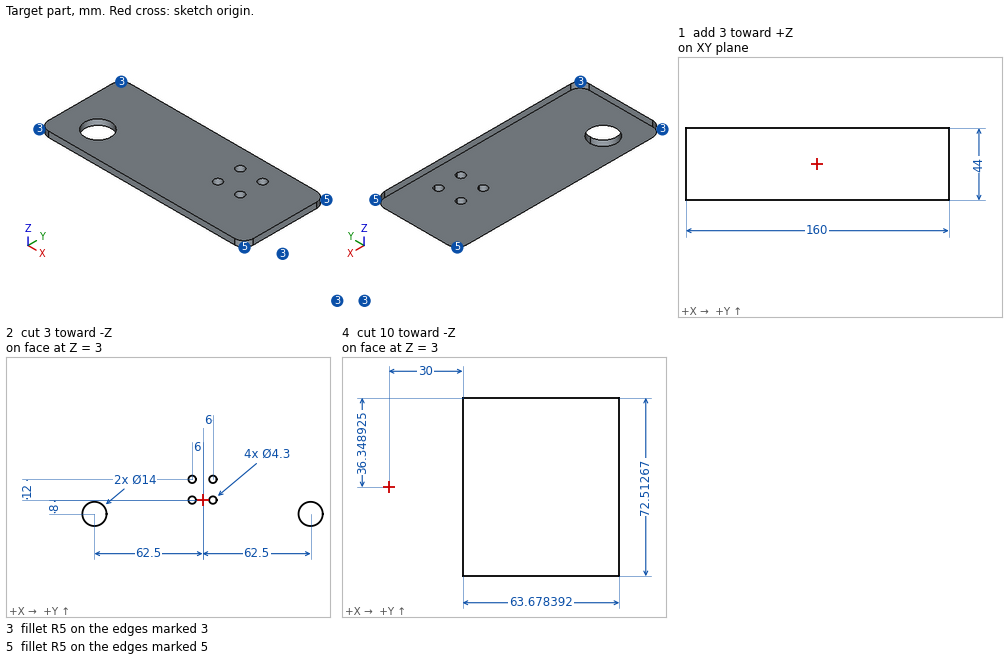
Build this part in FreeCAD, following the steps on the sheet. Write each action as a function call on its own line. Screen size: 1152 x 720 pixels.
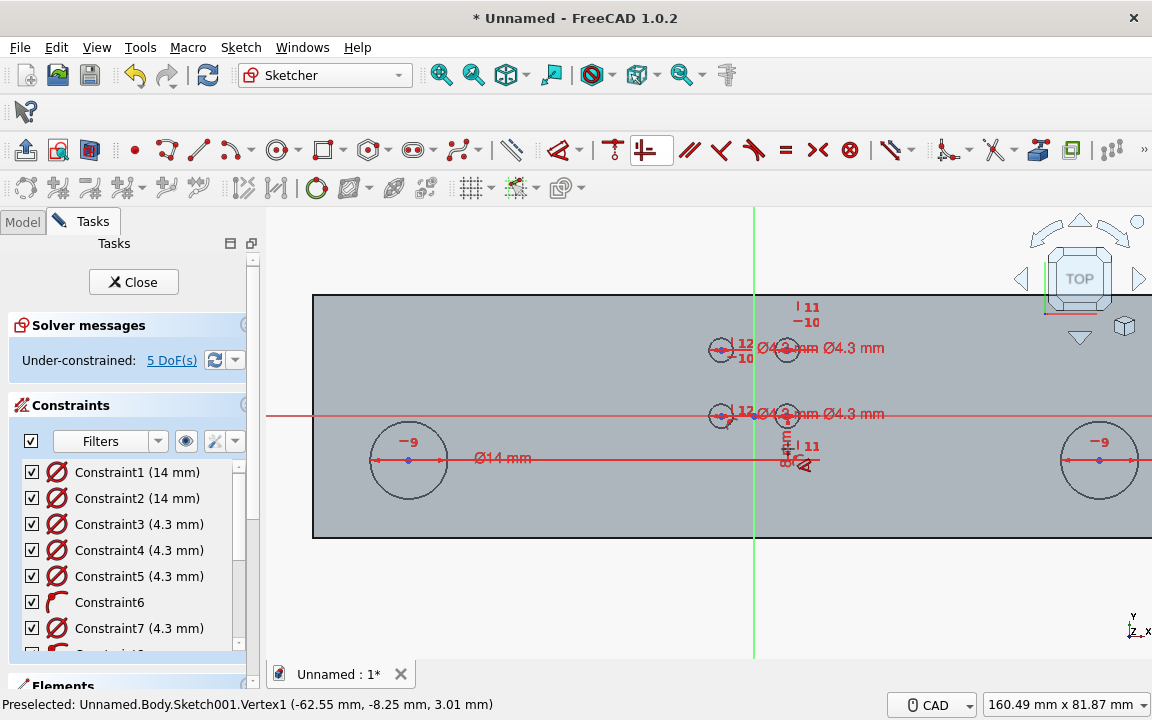
click(721, 350)
click(738, 316)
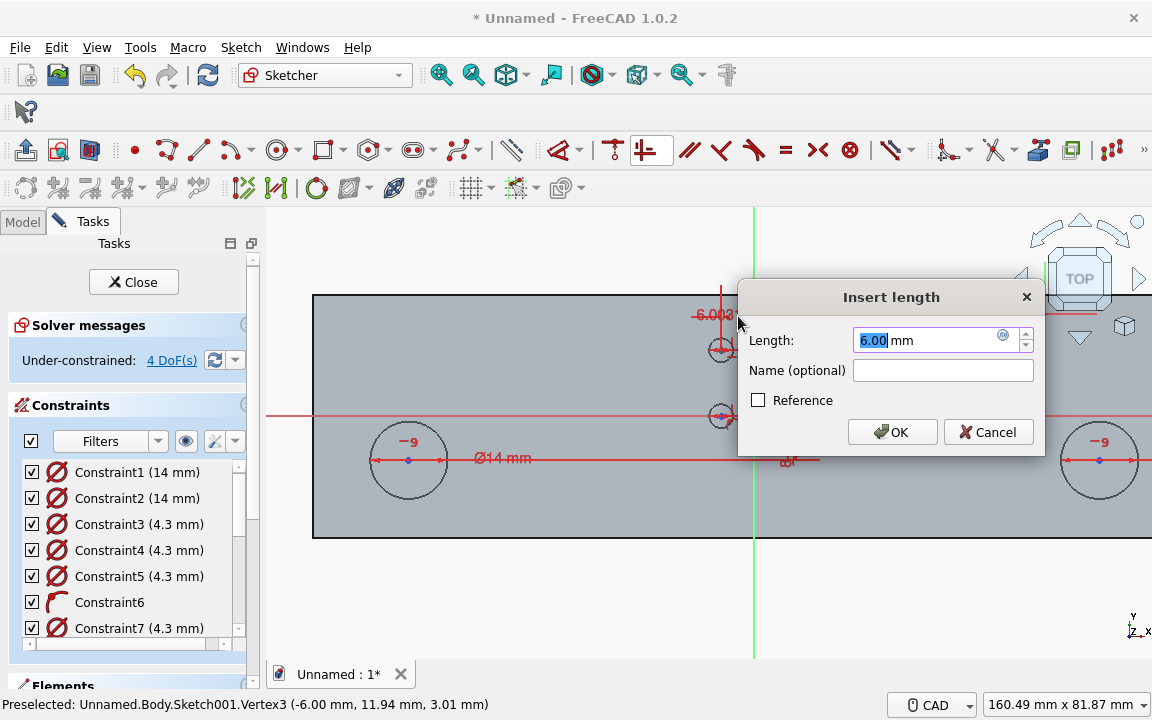
text(6)
key(Return)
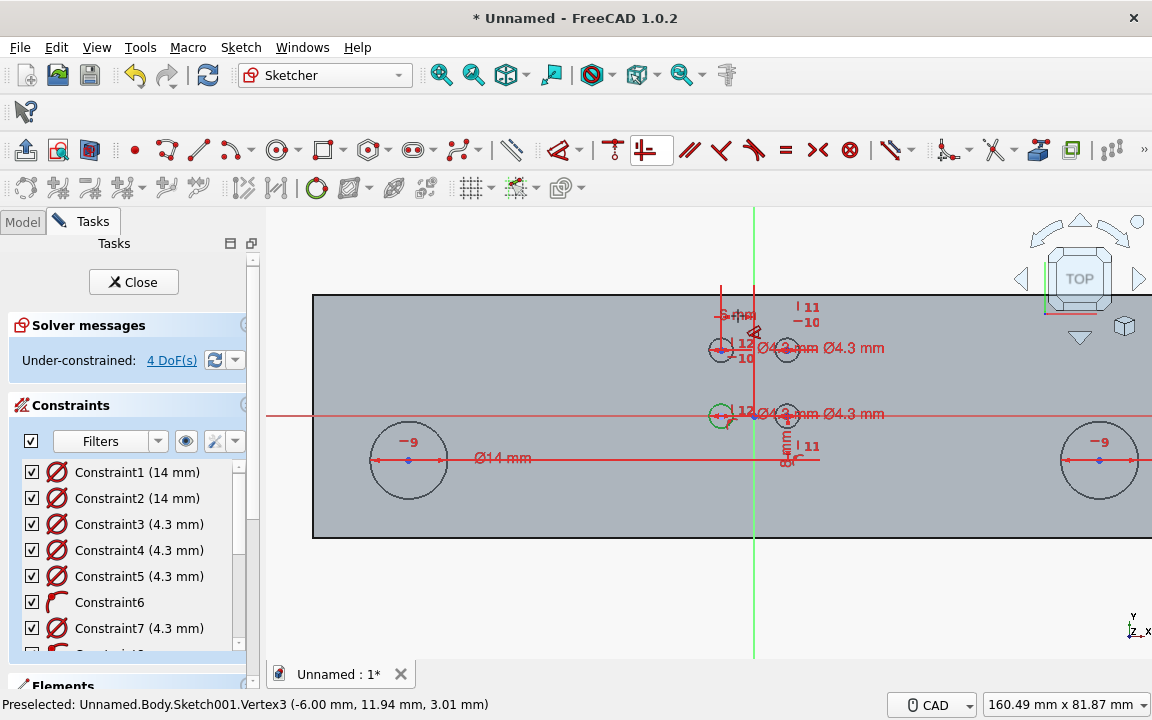
click(787, 350)
click(771, 292)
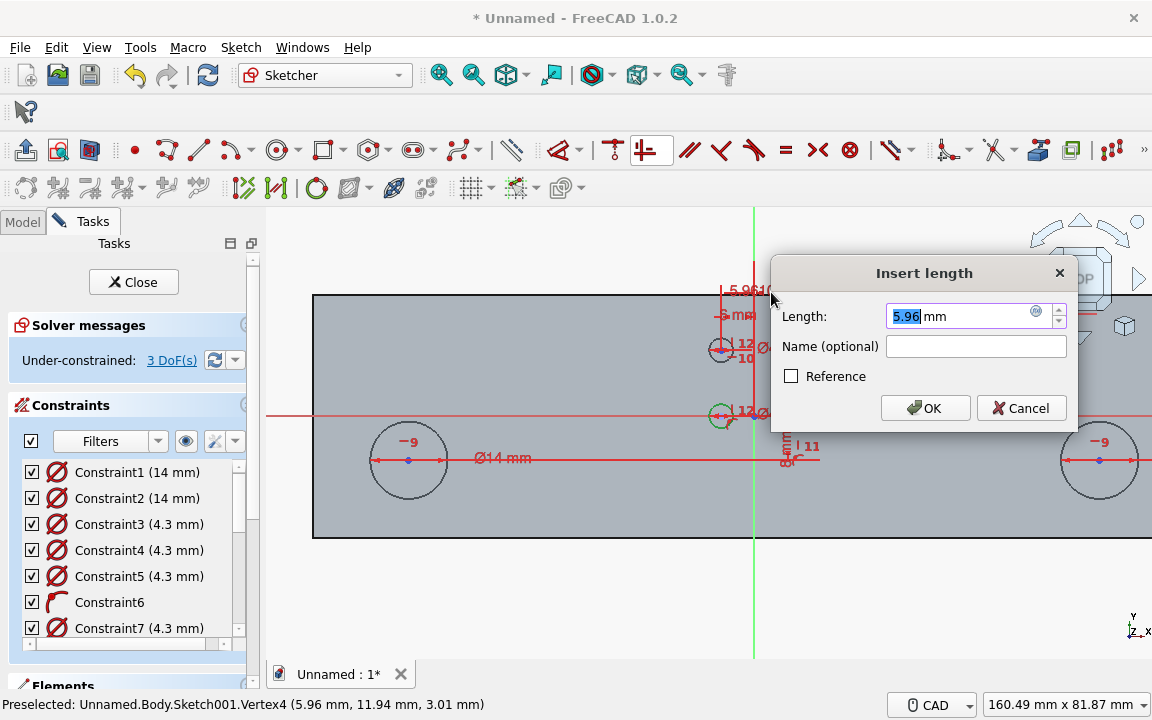
text(6)
key(Return)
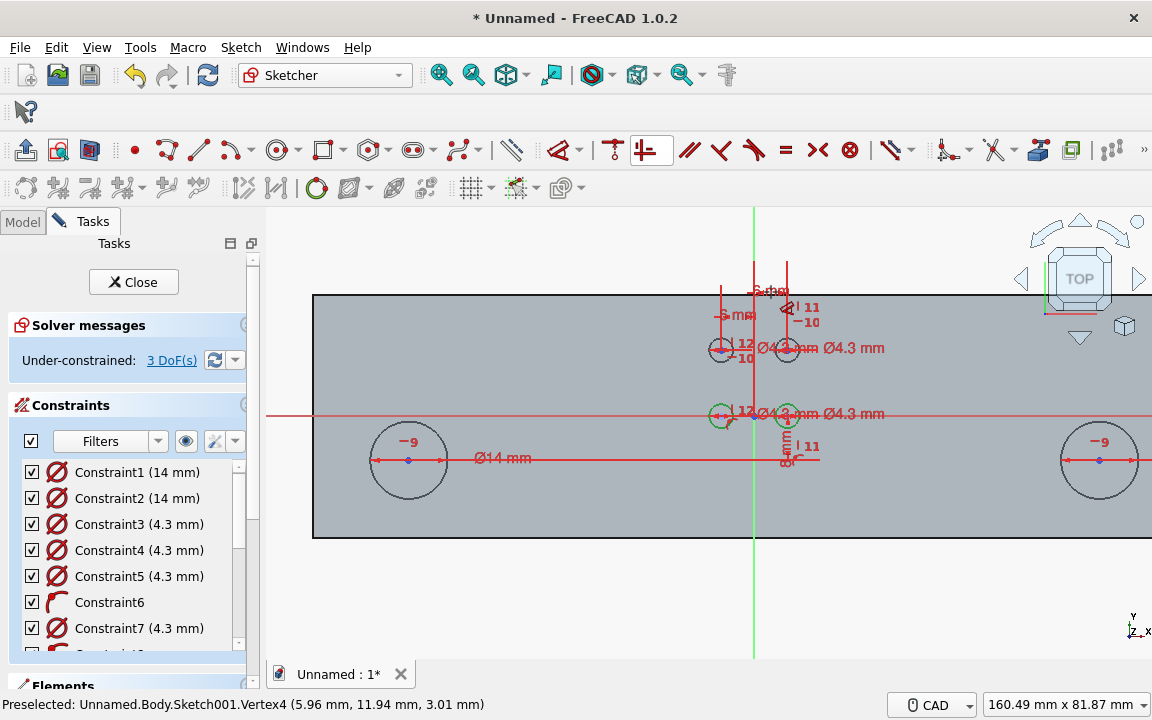
click(721, 350)
click(687, 383)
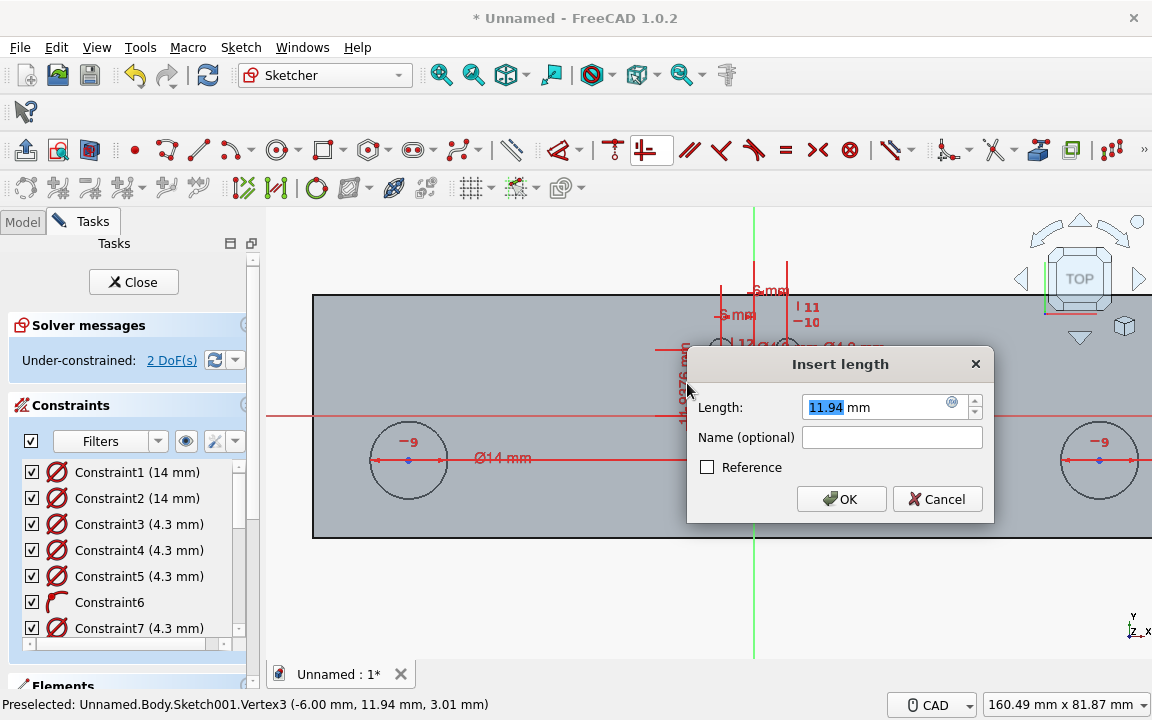
text(12)
key(Return)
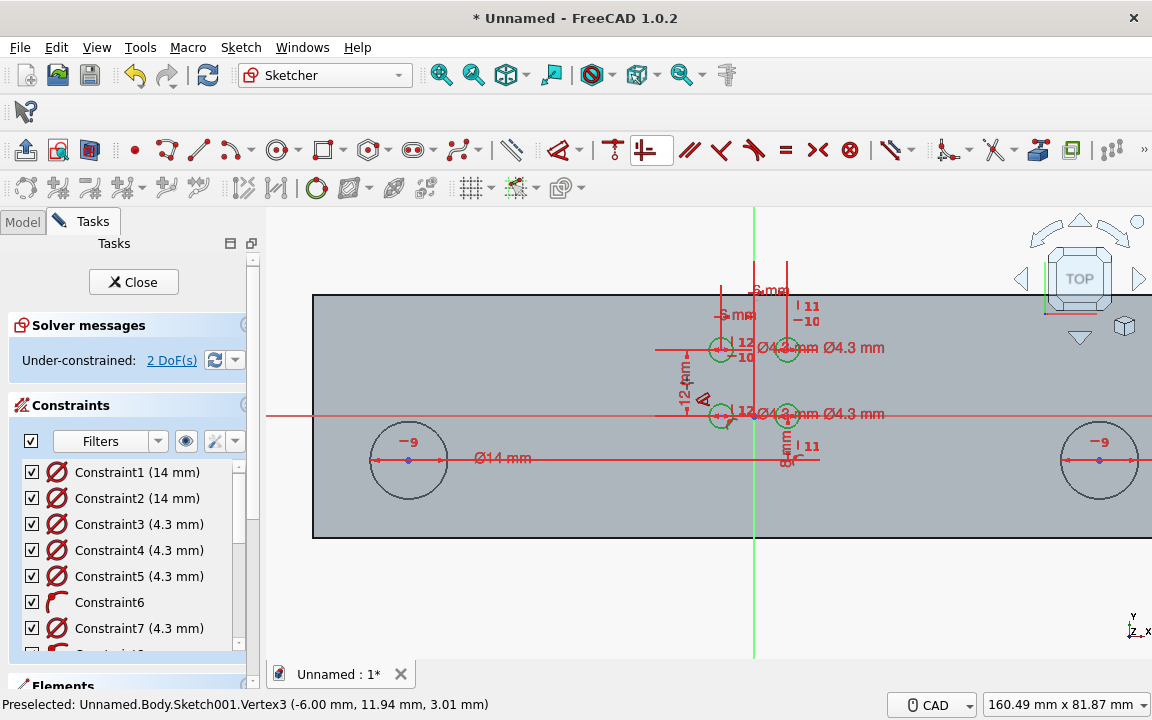
click(409, 460)
click(582, 494)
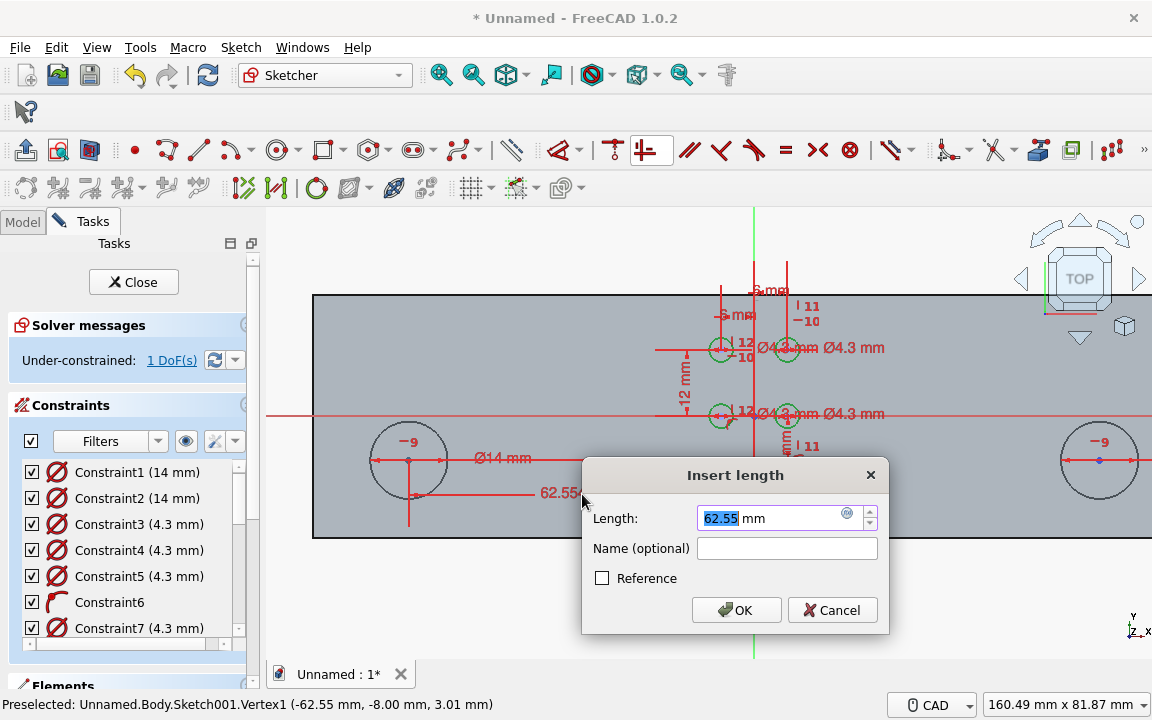
text(62.5)
key(Return)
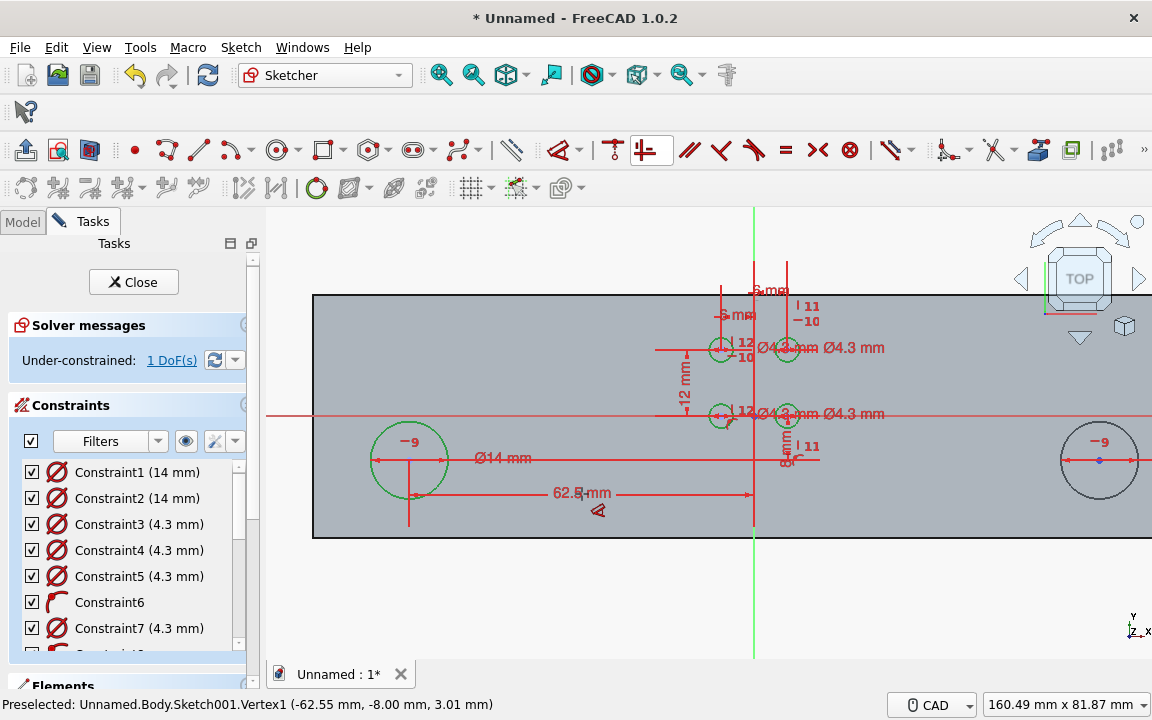
scroll(409, 462, down, 2)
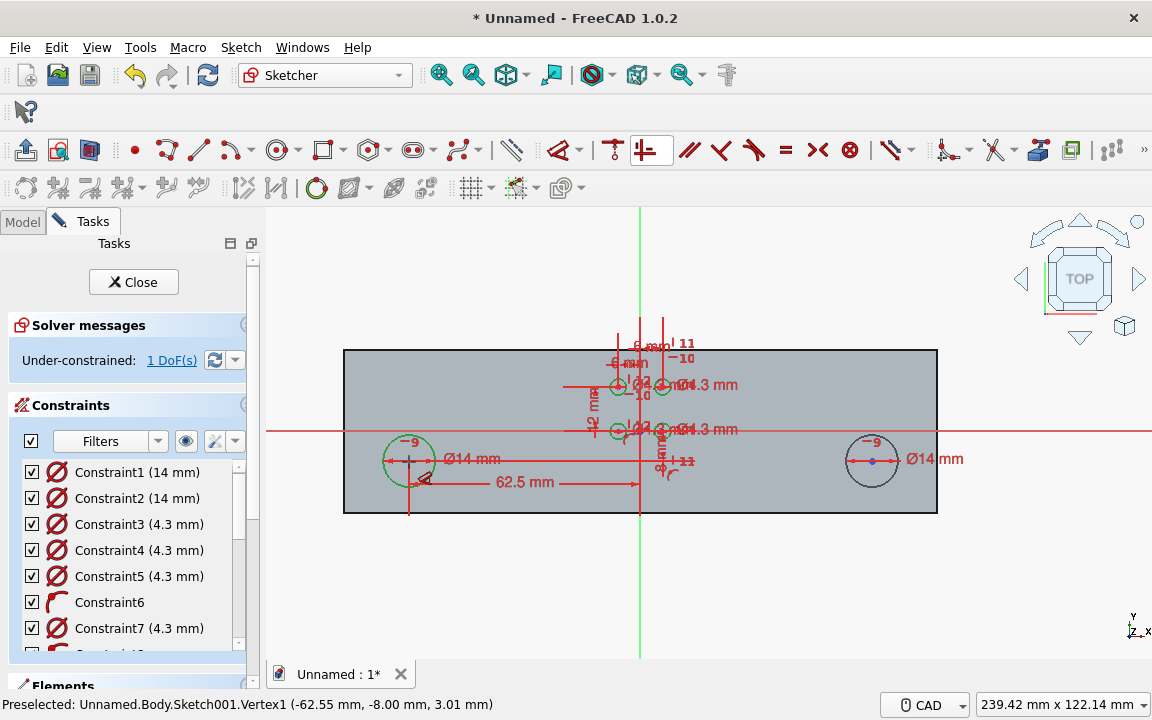
click(872, 461)
click(756, 495)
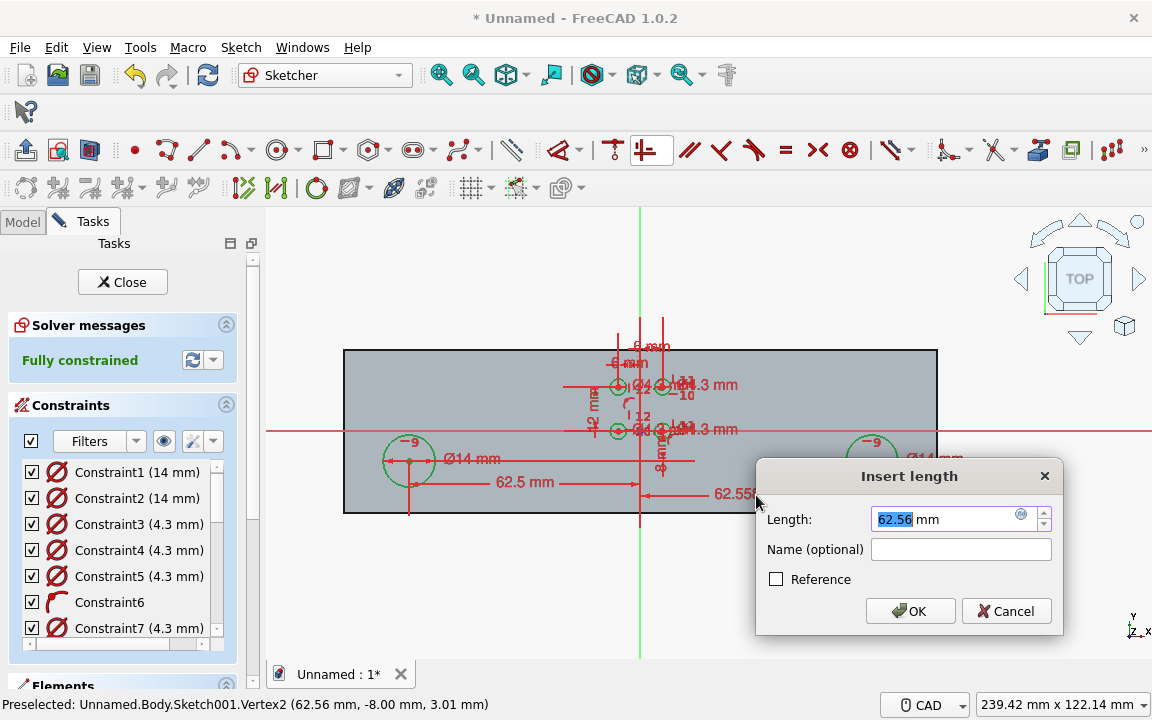
text(62.5)
key(Return)
key(Escape)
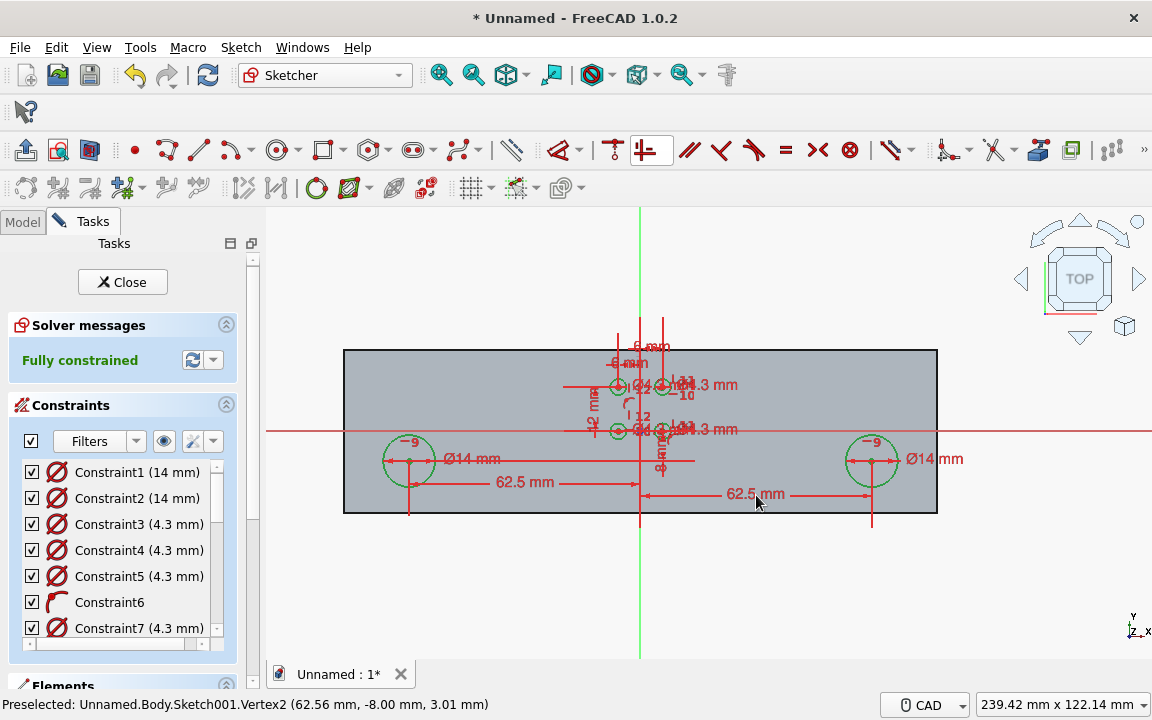
click(123, 282)